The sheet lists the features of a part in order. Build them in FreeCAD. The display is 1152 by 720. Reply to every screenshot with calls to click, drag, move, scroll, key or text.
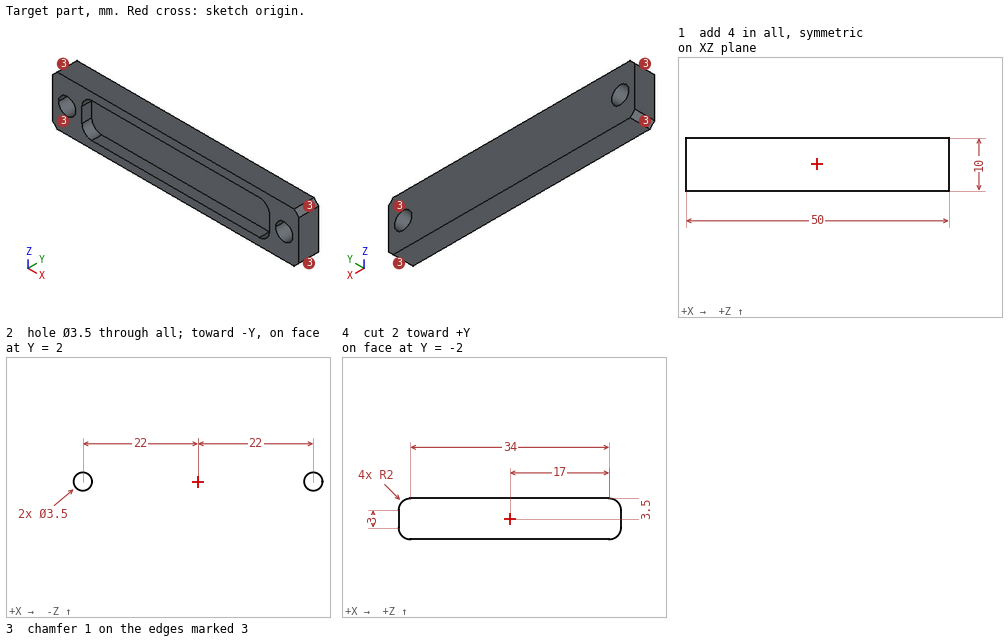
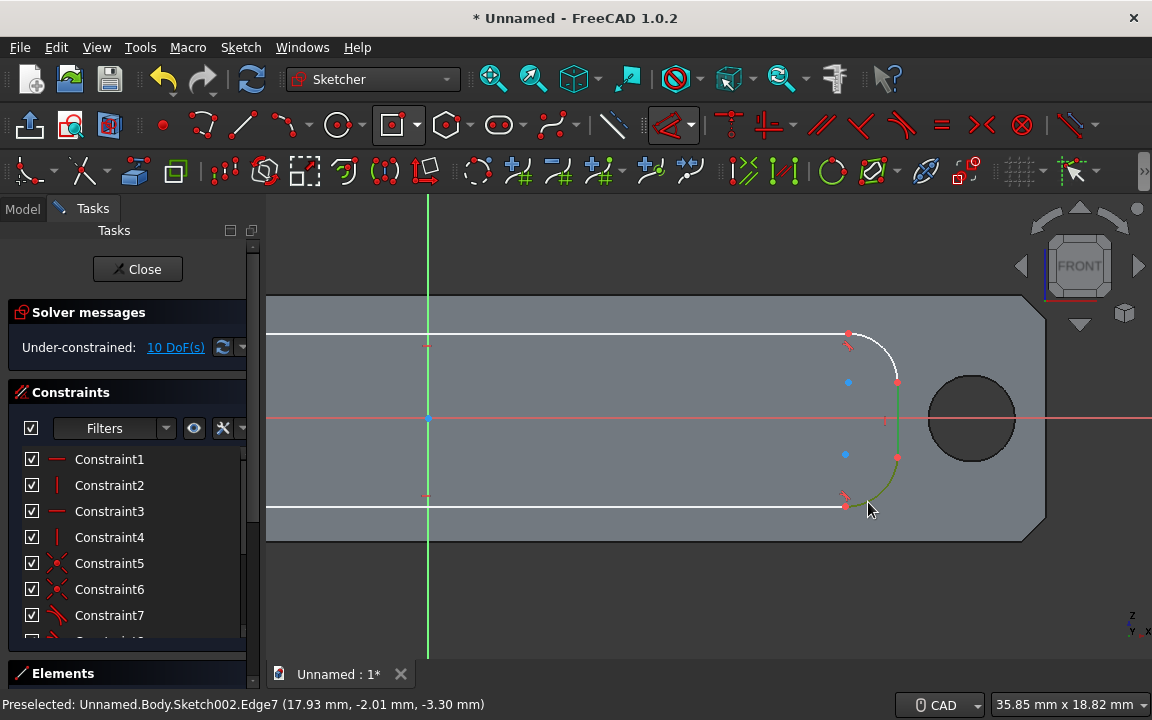
click(902, 126)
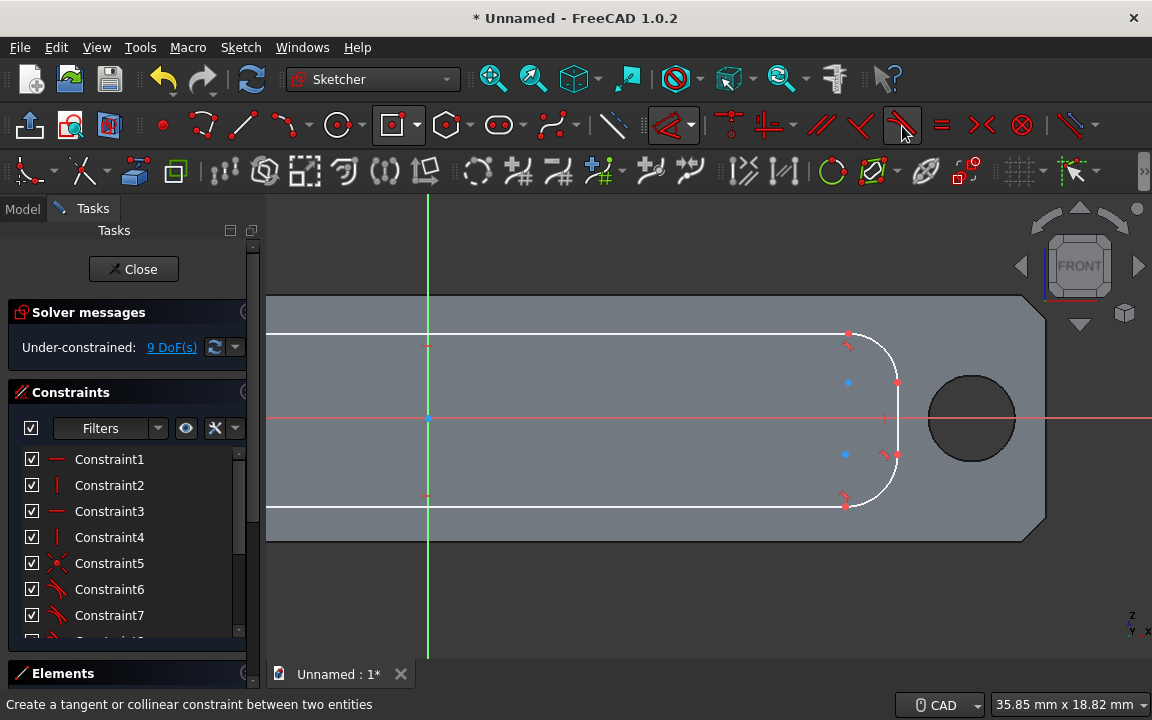
click(898, 433)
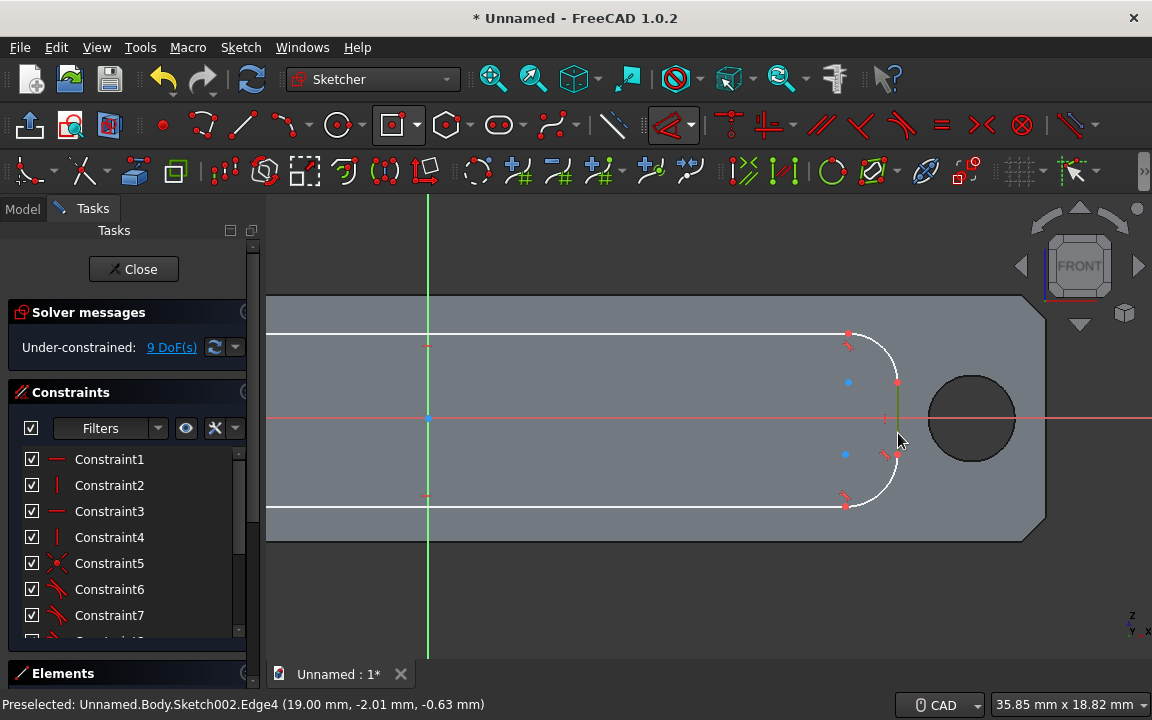
click(892, 361)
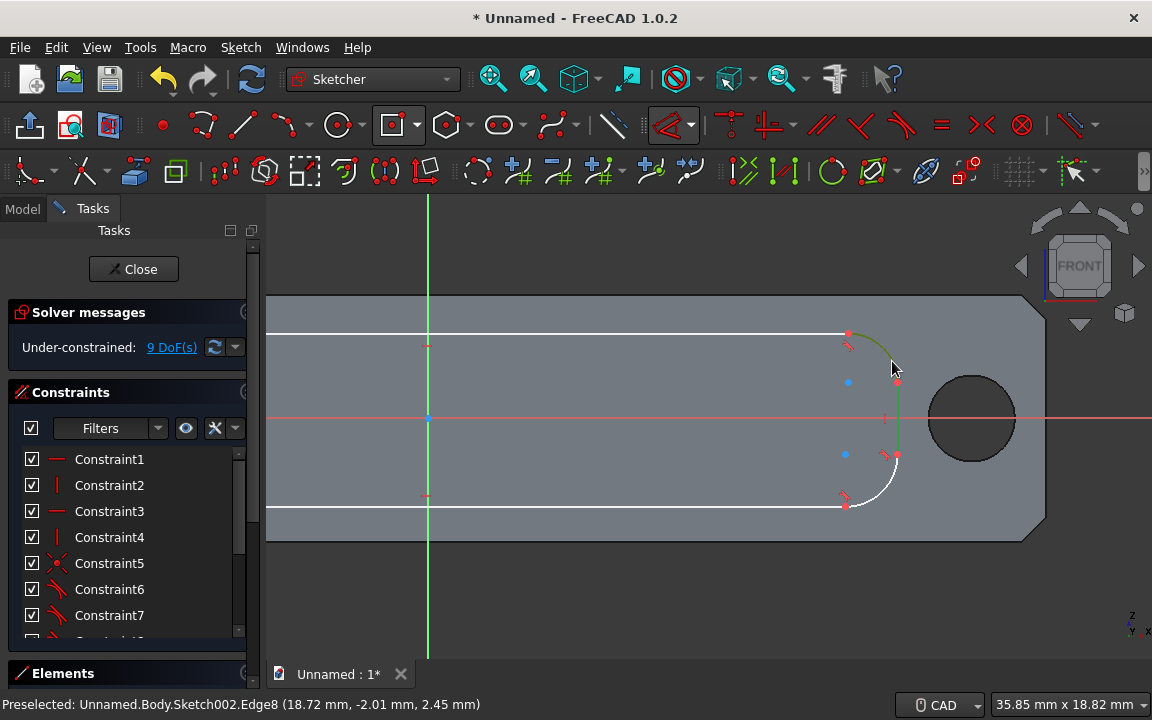
click(902, 126)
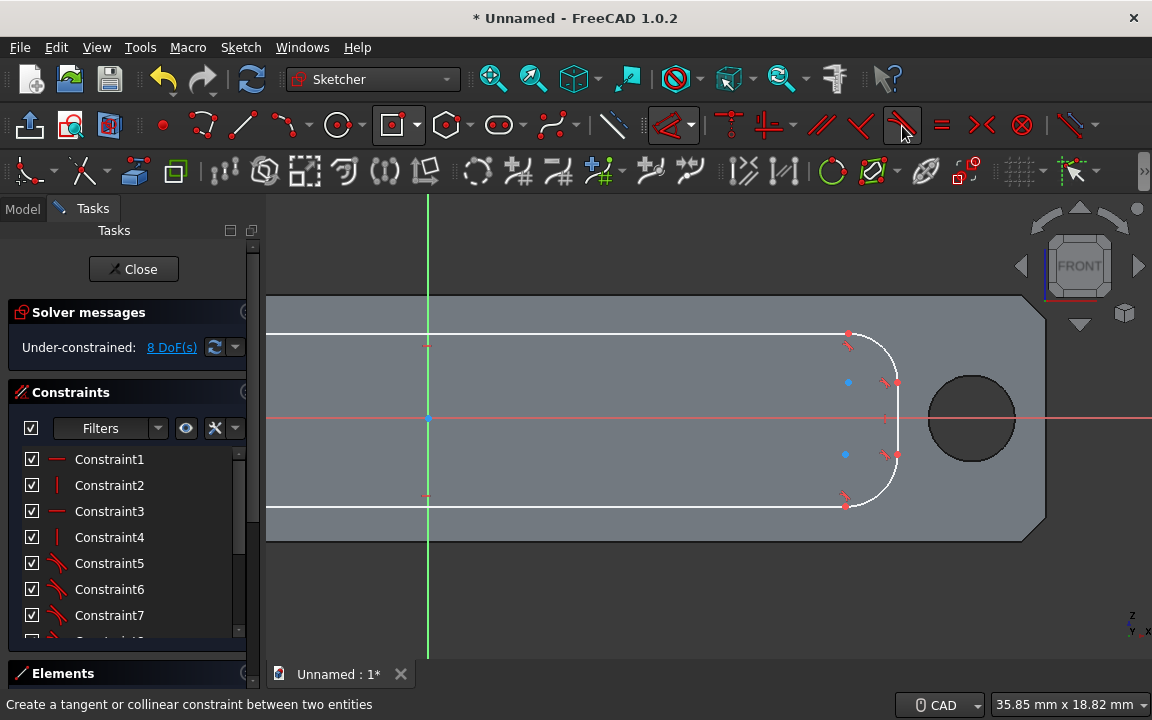
scroll(899, 436, down, 3)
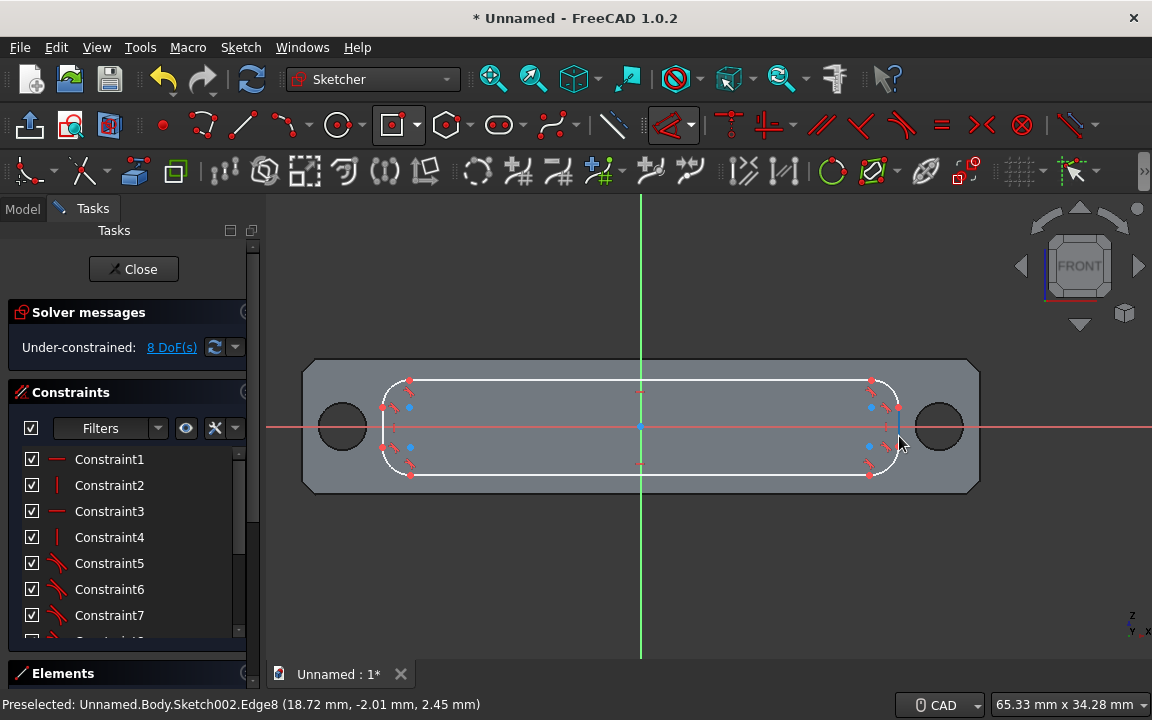
click(398, 383)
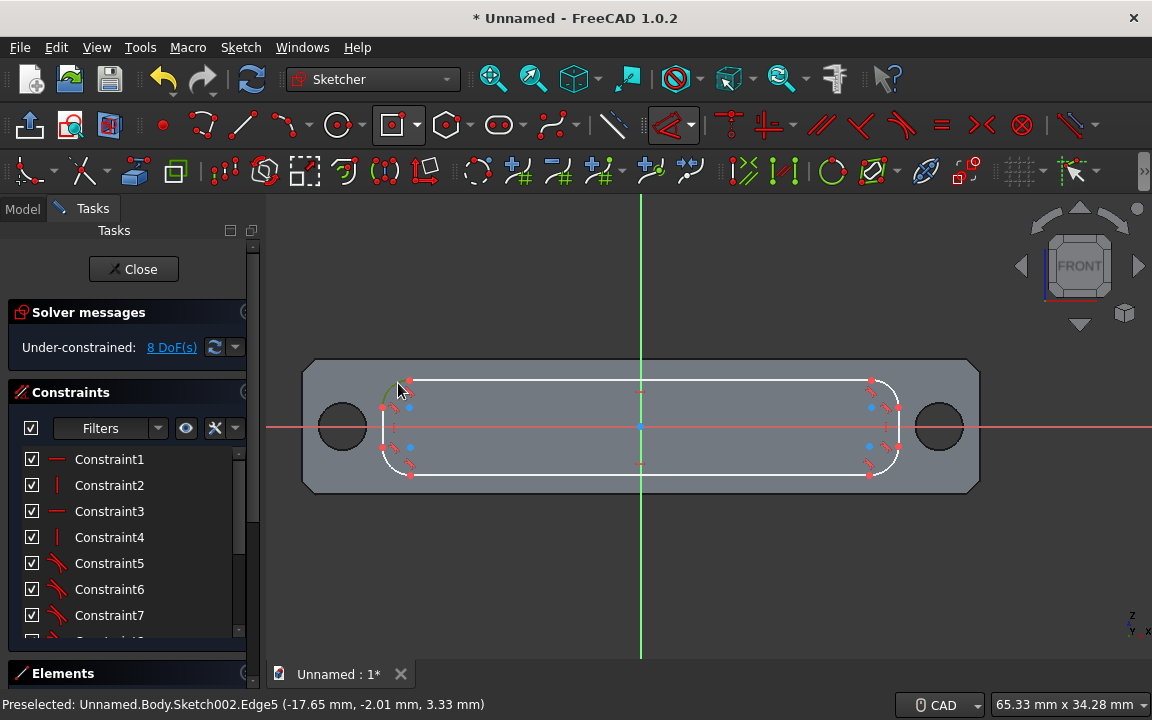
click(386, 460)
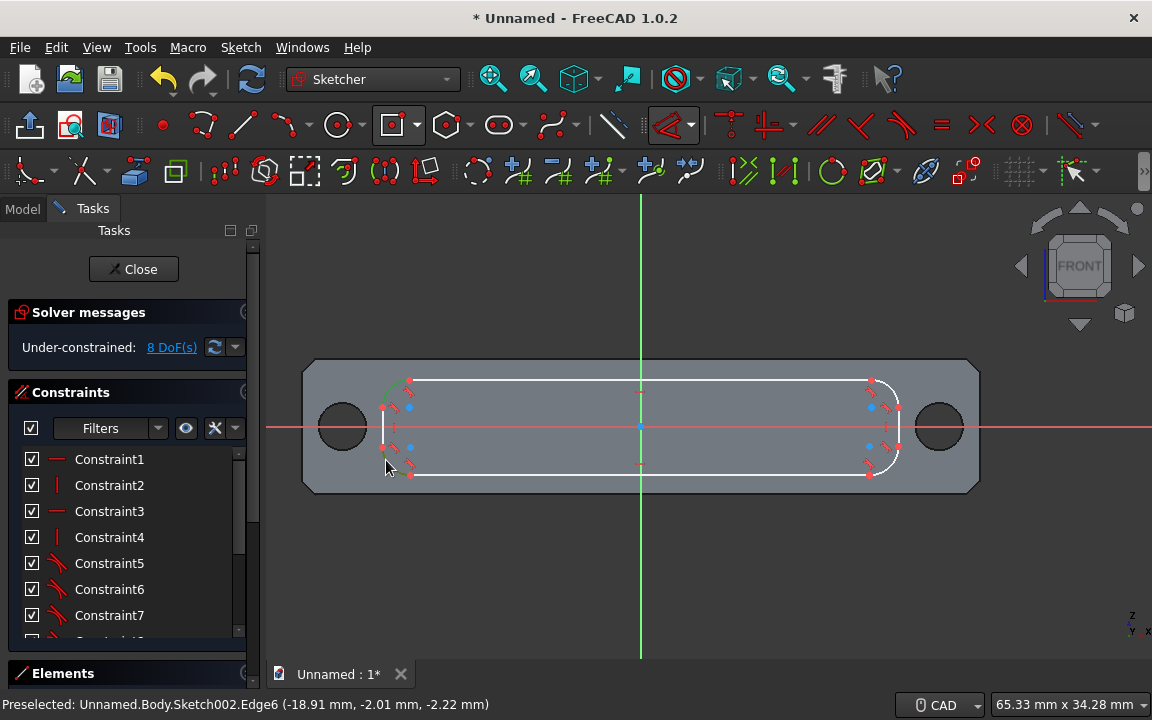
click(883, 472)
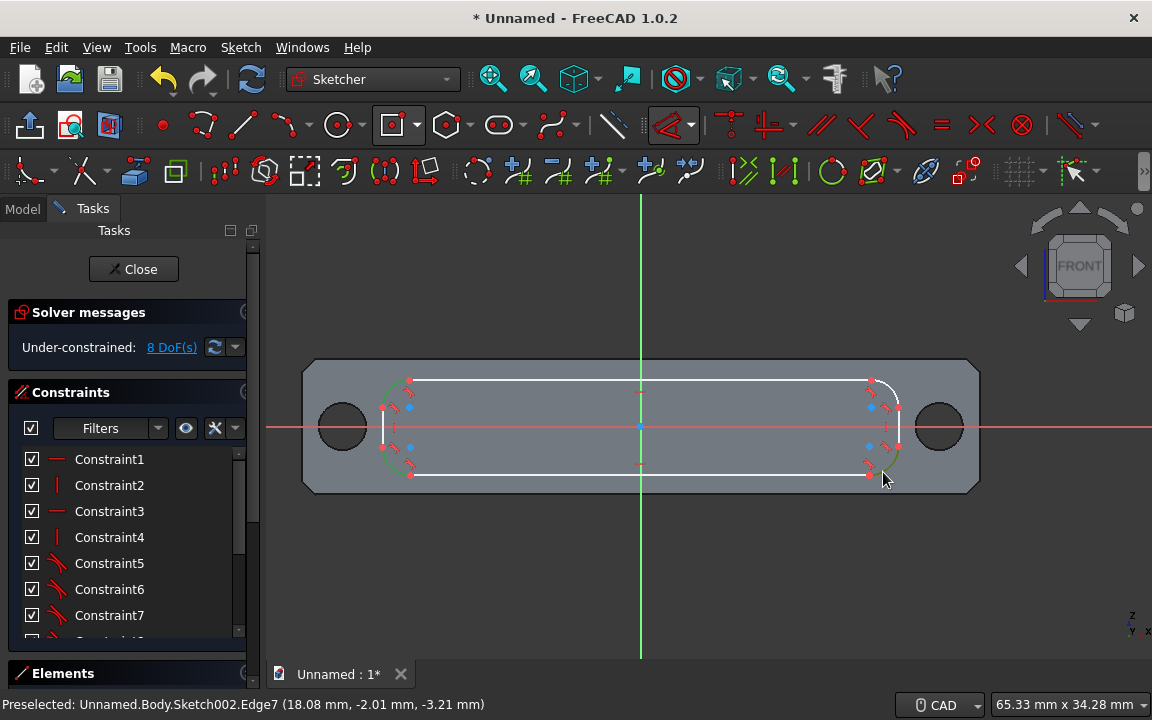
click(896, 395)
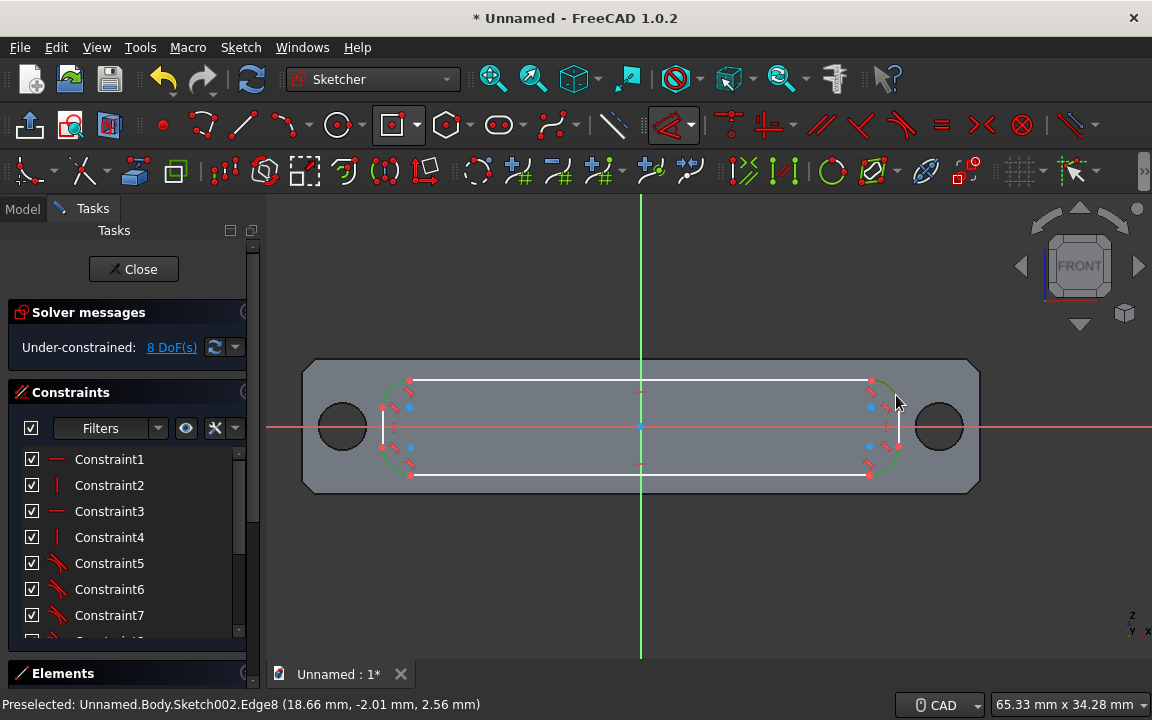
click(942, 126)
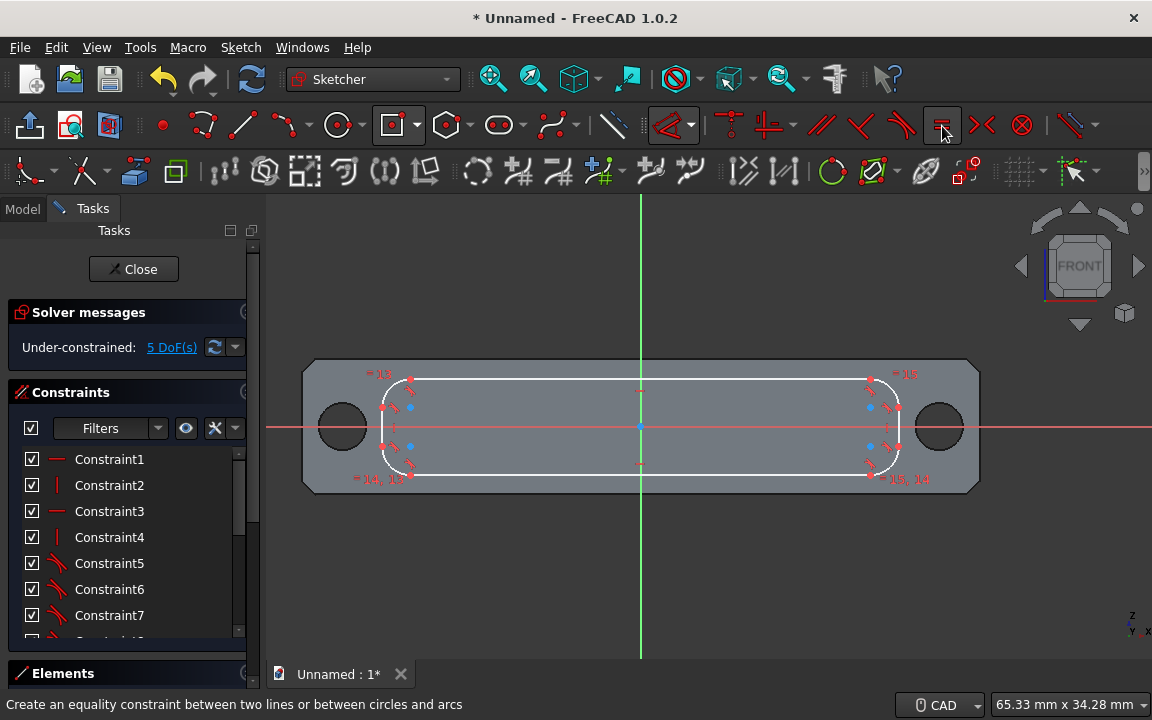
scroll(398, 382, up, 2)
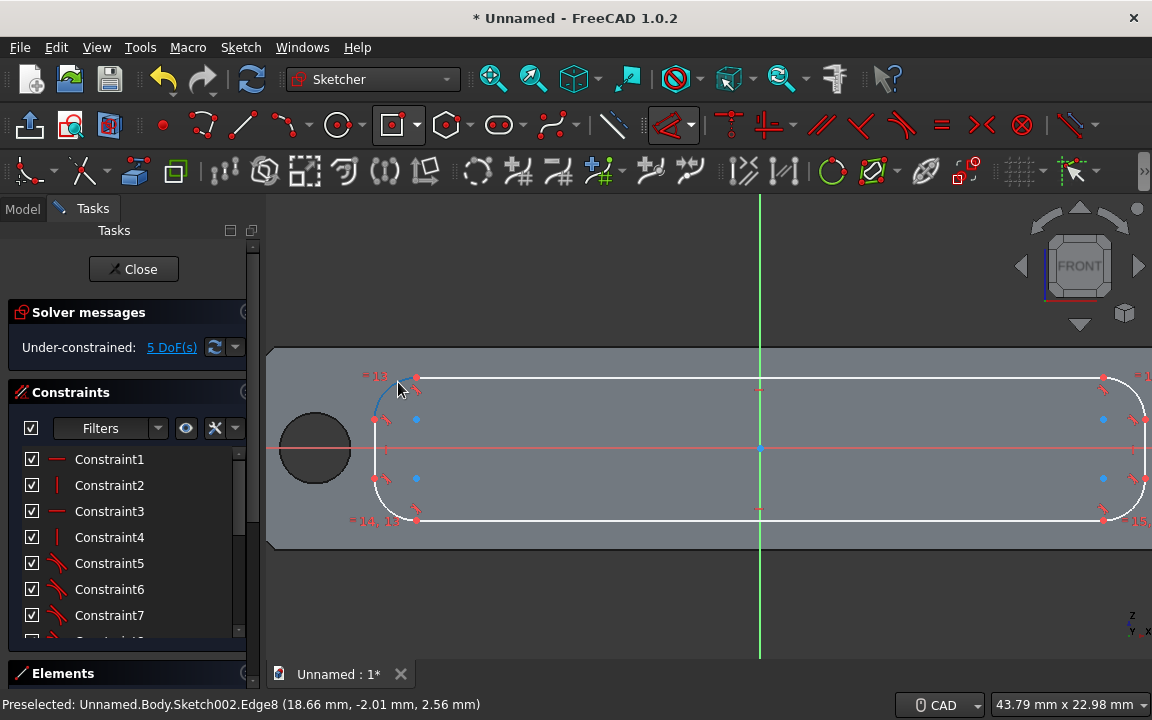
click(398, 382)